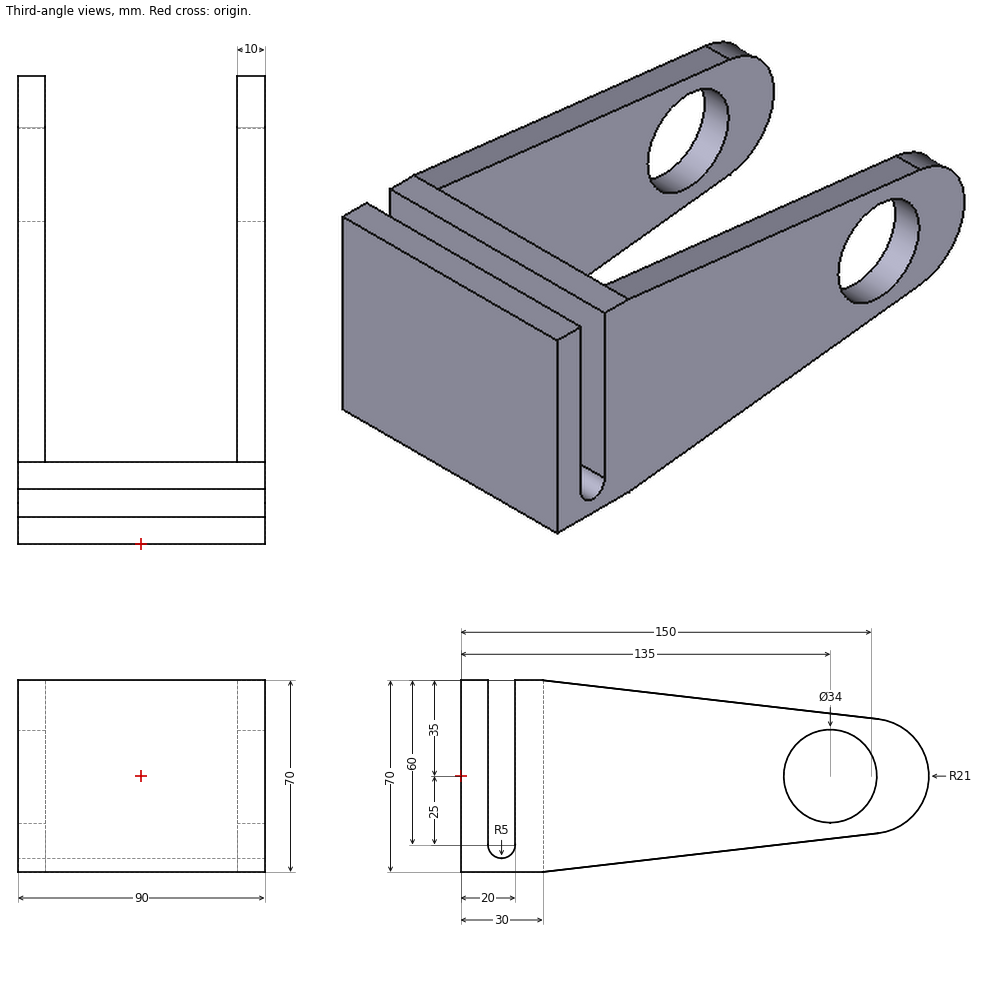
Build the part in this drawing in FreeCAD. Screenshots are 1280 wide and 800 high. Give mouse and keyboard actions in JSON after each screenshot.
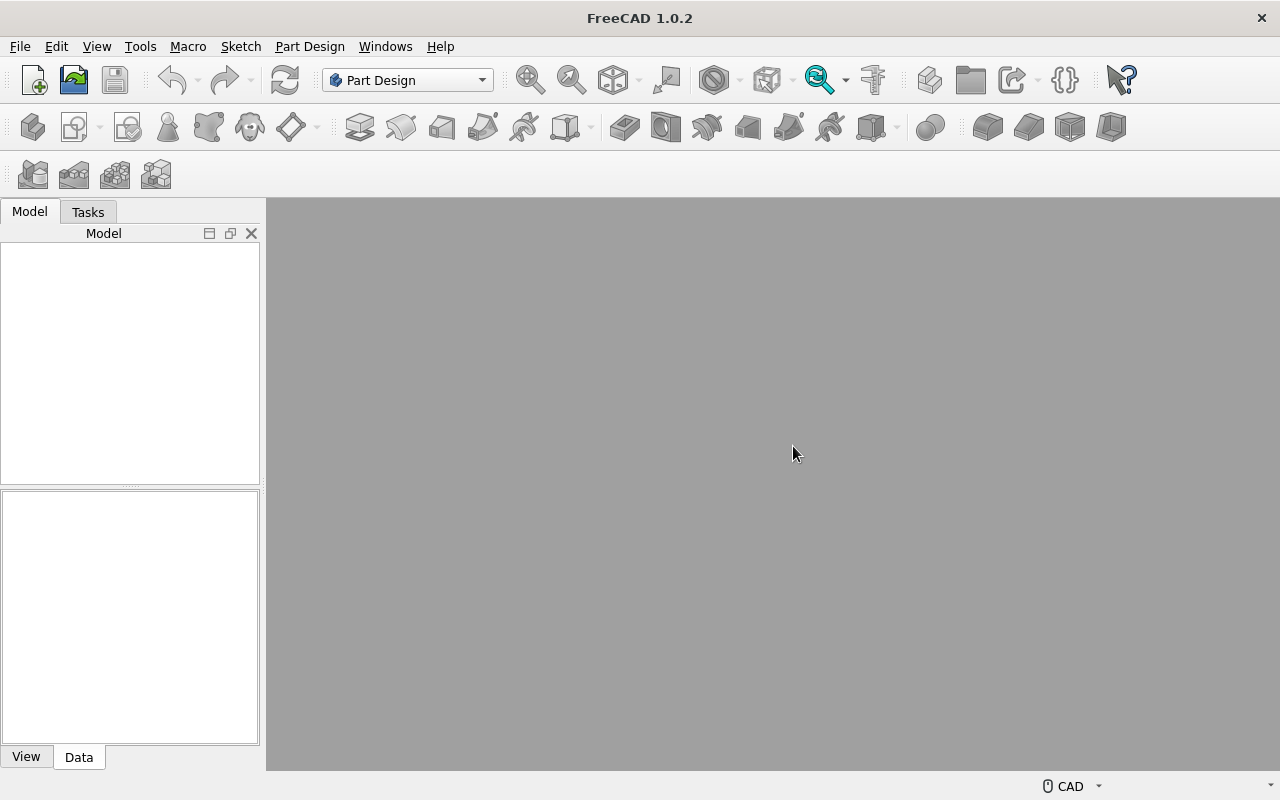
{"action": "left_click", "coordinate": [33, 80]}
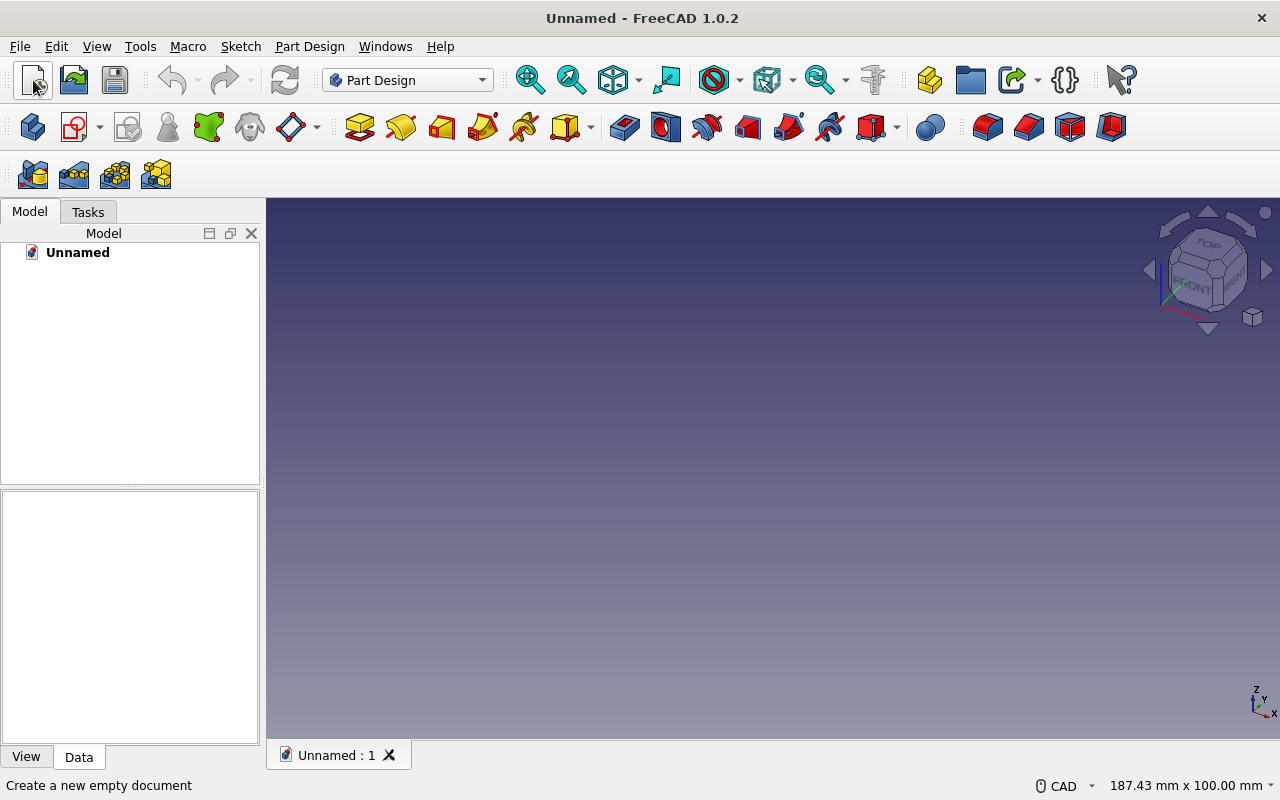
{"action": "left_click", "coordinate": [74, 128]}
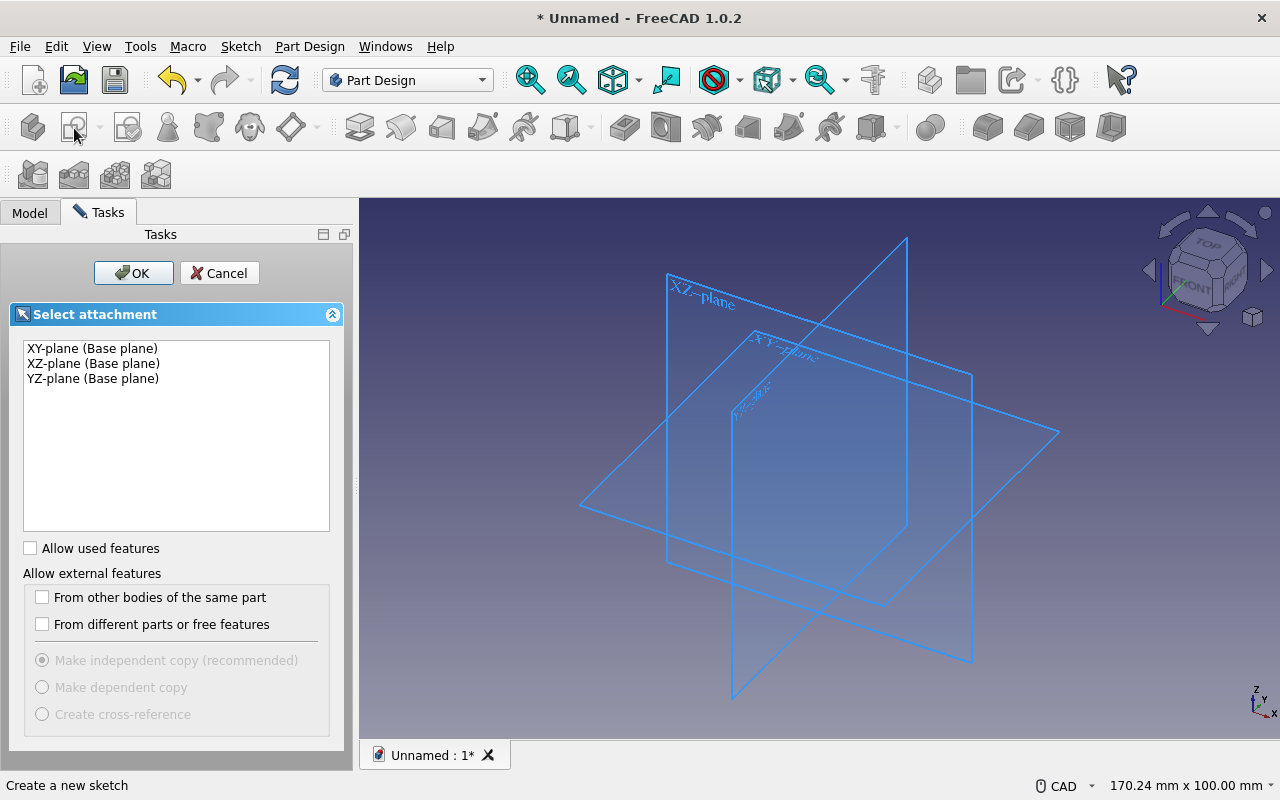
{"action": "left_click", "coordinate": [84, 364]}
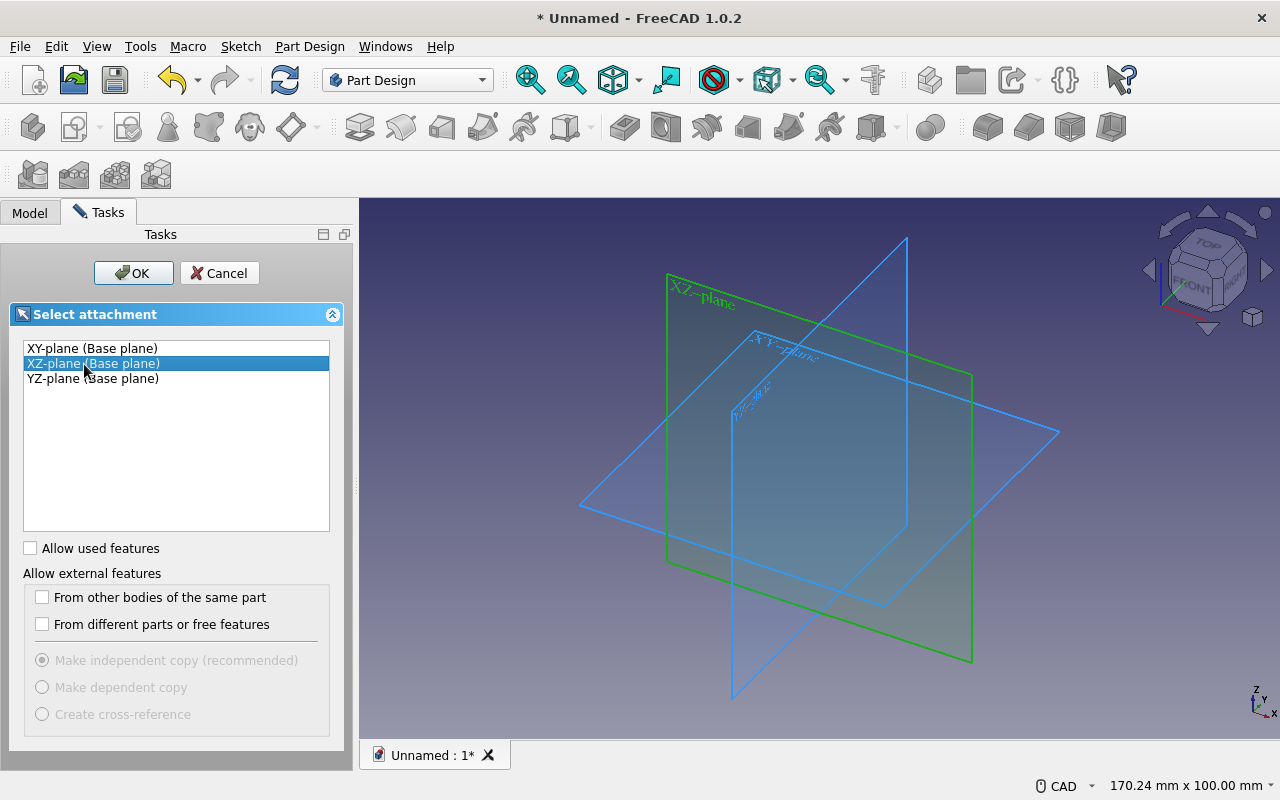
{"action": "left_click", "coordinate": [134, 273]}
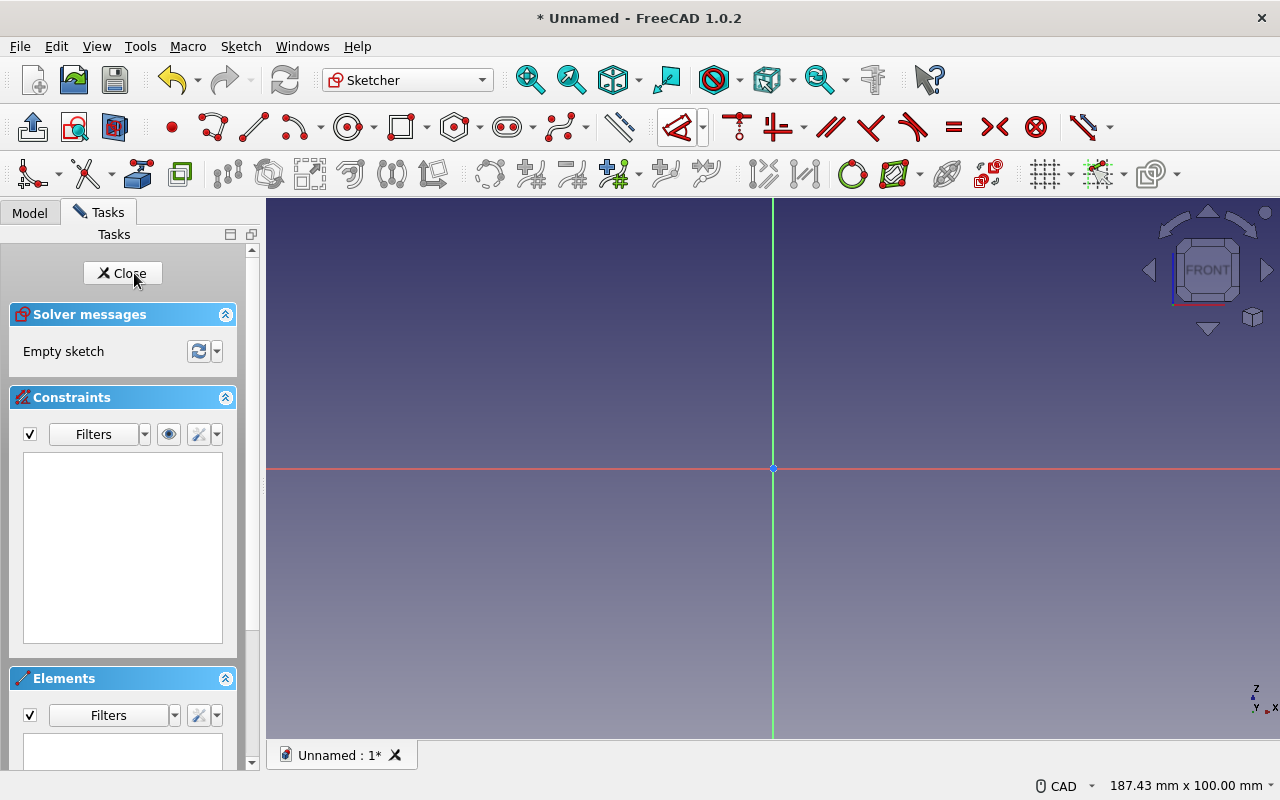
{"action": "left_click", "coordinate": [426, 128]}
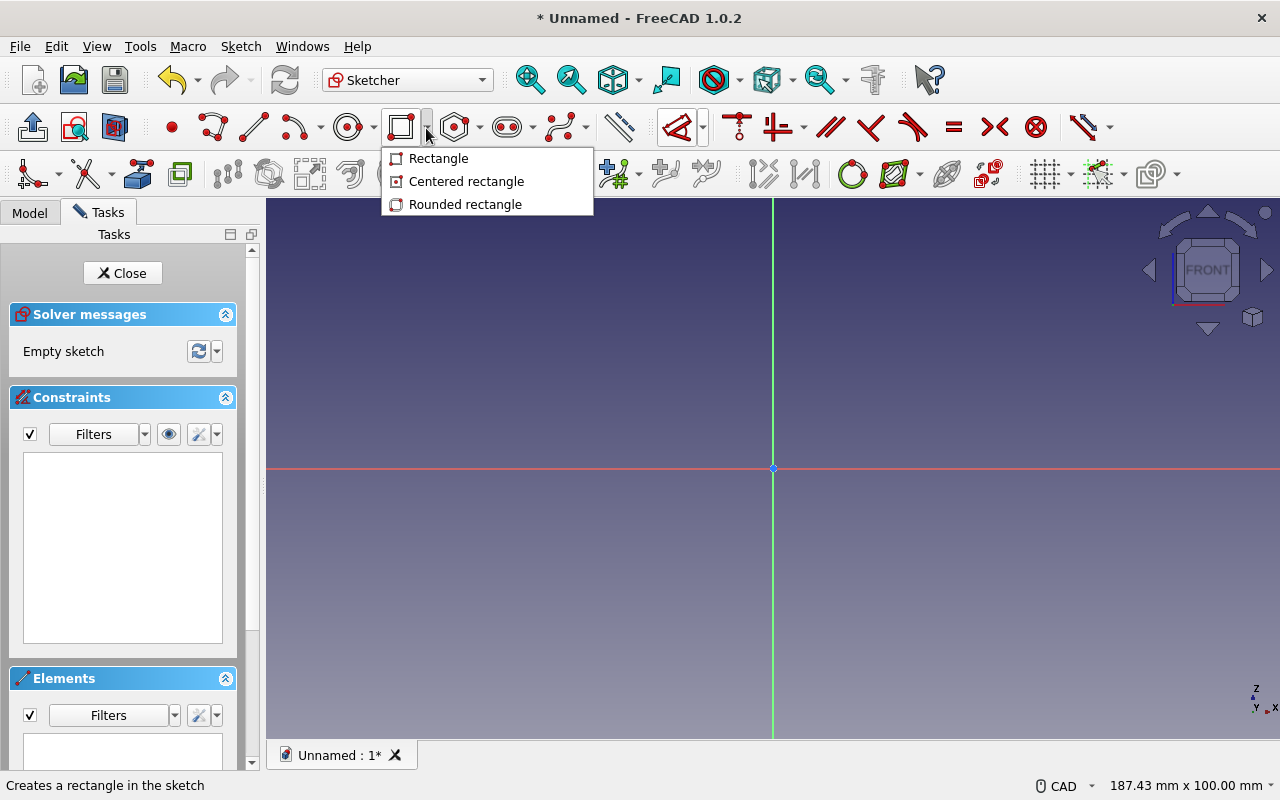
{"action": "left_click", "coordinate": [488, 182]}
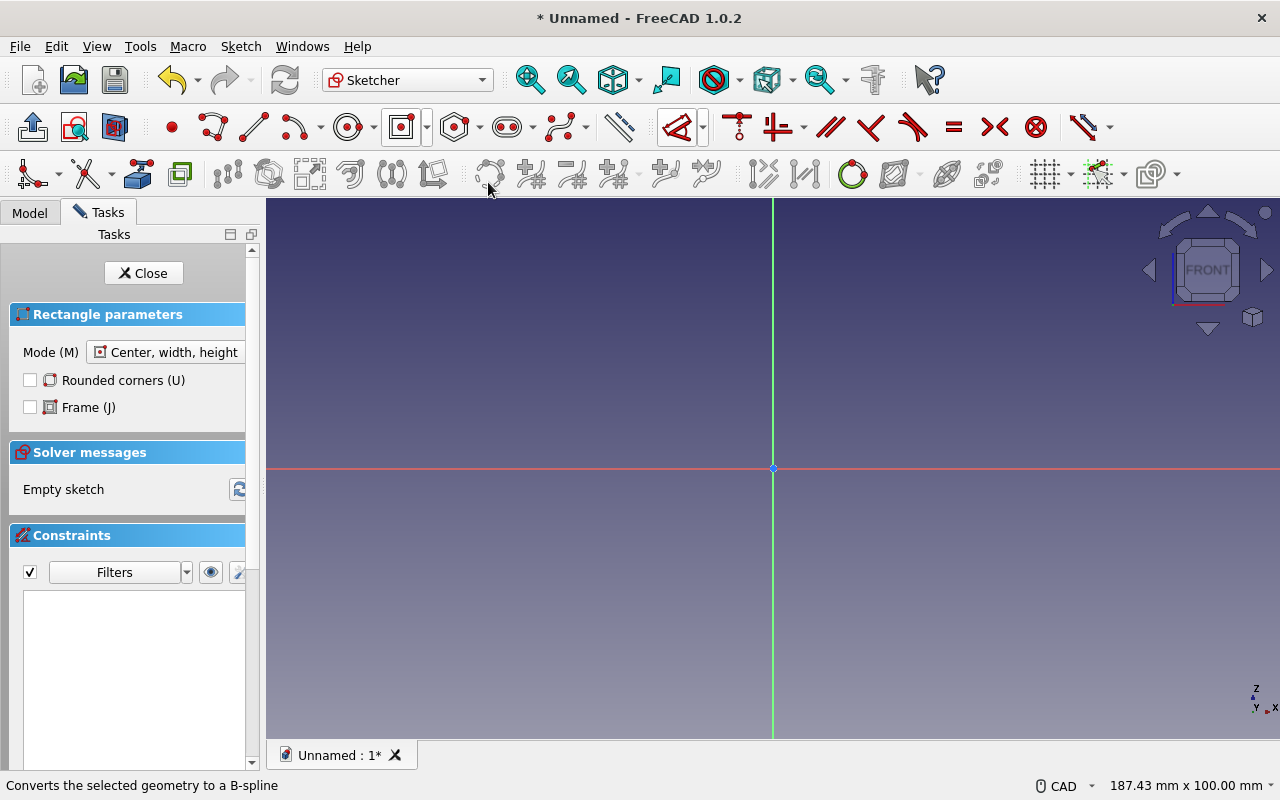
{"action": "left_click", "coordinate": [773, 468]}
{"action": "left_click", "coordinate": [1016, 279]}
{"action": "key", "text": "Escape"}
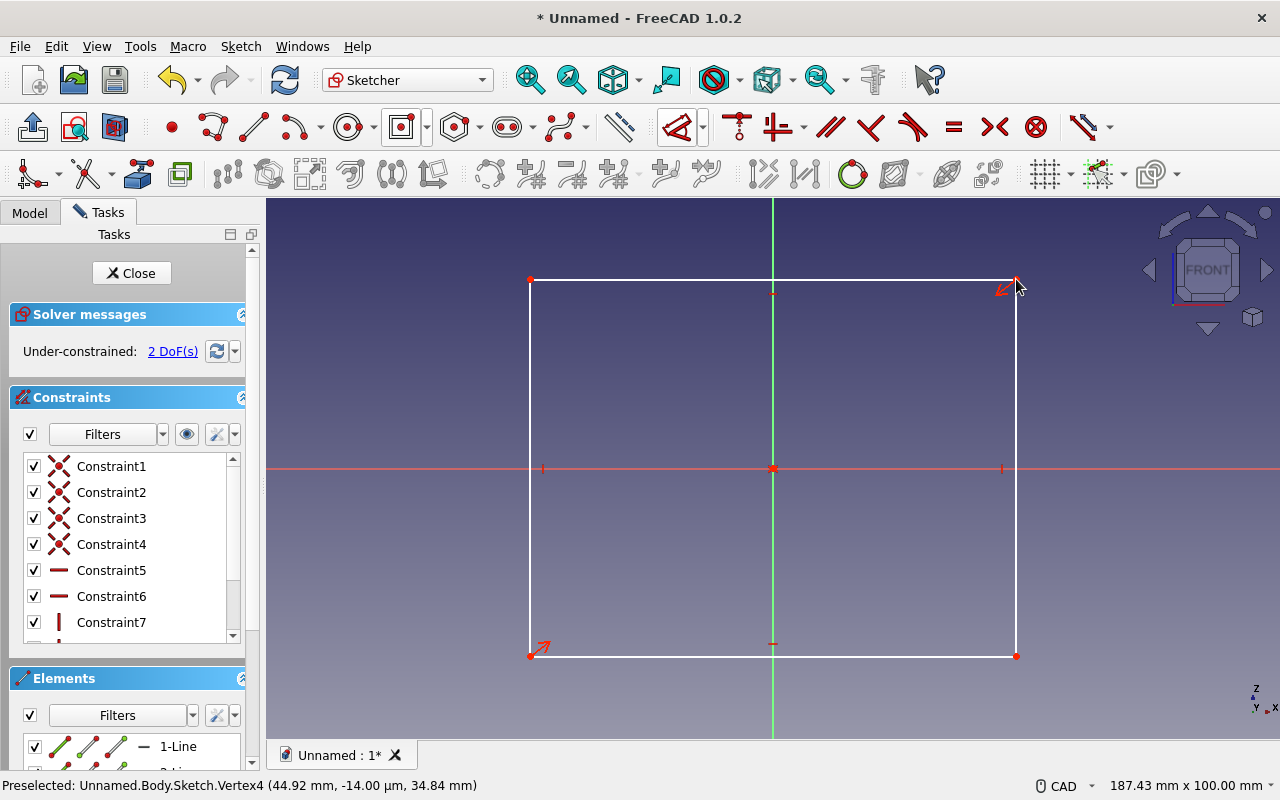
{"action": "left_click", "coordinate": [676, 128]}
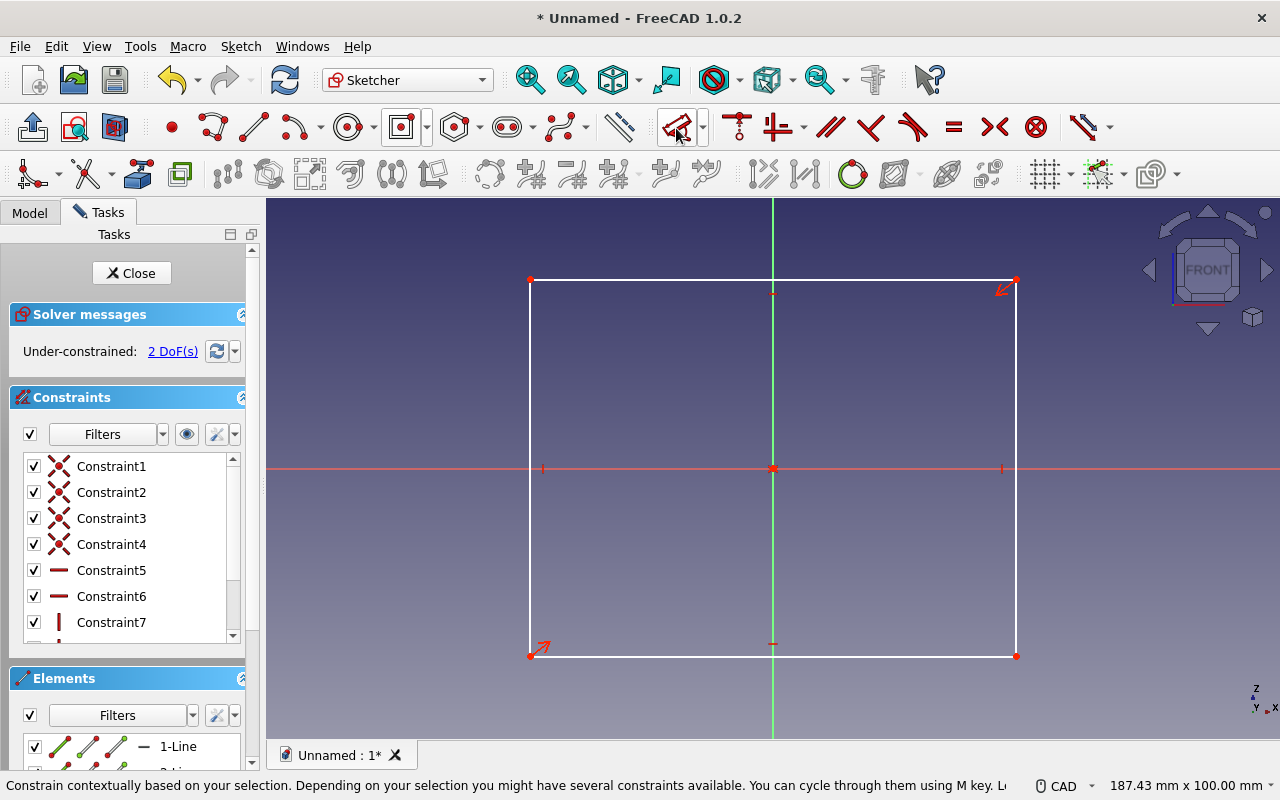
{"action": "left_click", "coordinate": [676, 657]}
{"action": "left_click", "coordinate": [661, 691]}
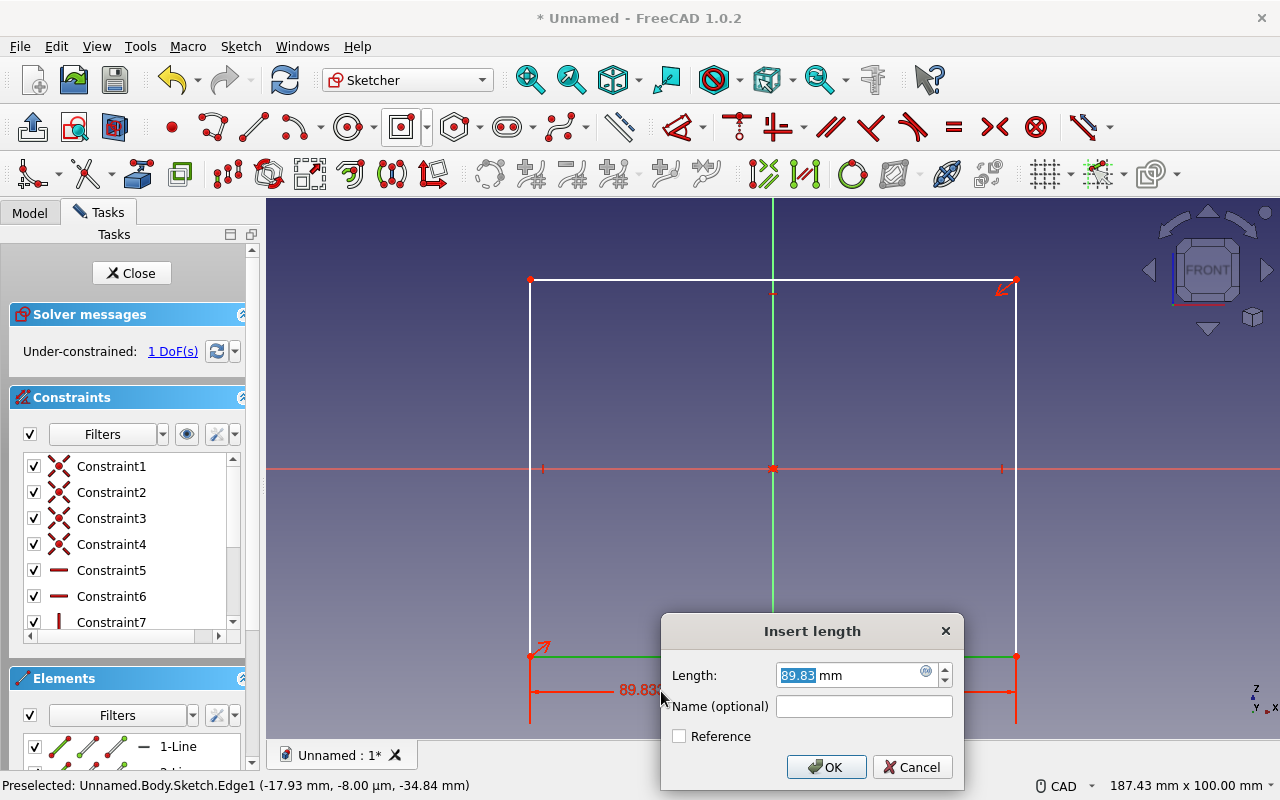
{"action": "type", "text": "90"}
{"action": "key", "text": "Return"}